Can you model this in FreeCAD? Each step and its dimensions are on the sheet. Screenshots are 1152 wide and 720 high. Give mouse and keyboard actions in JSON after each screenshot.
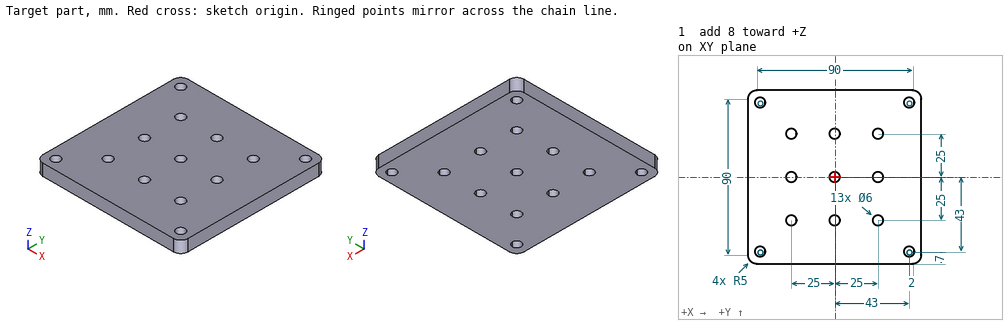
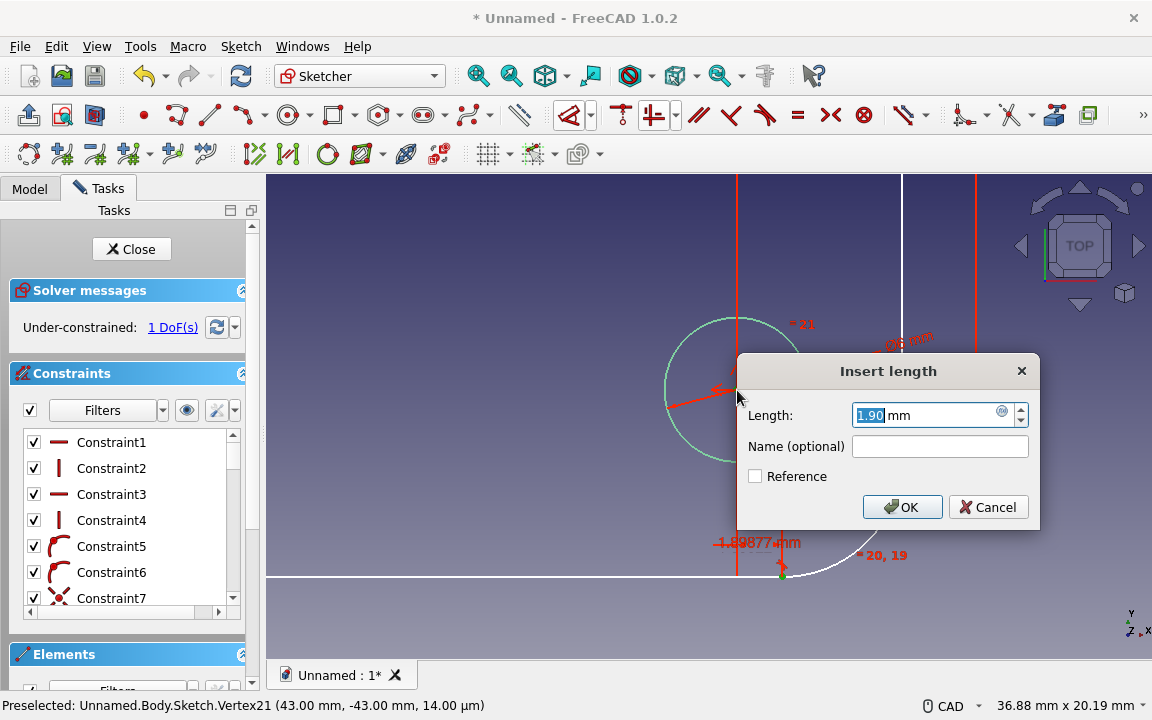
{"action": "type", "text": "2"}
{"action": "key", "text": "Return"}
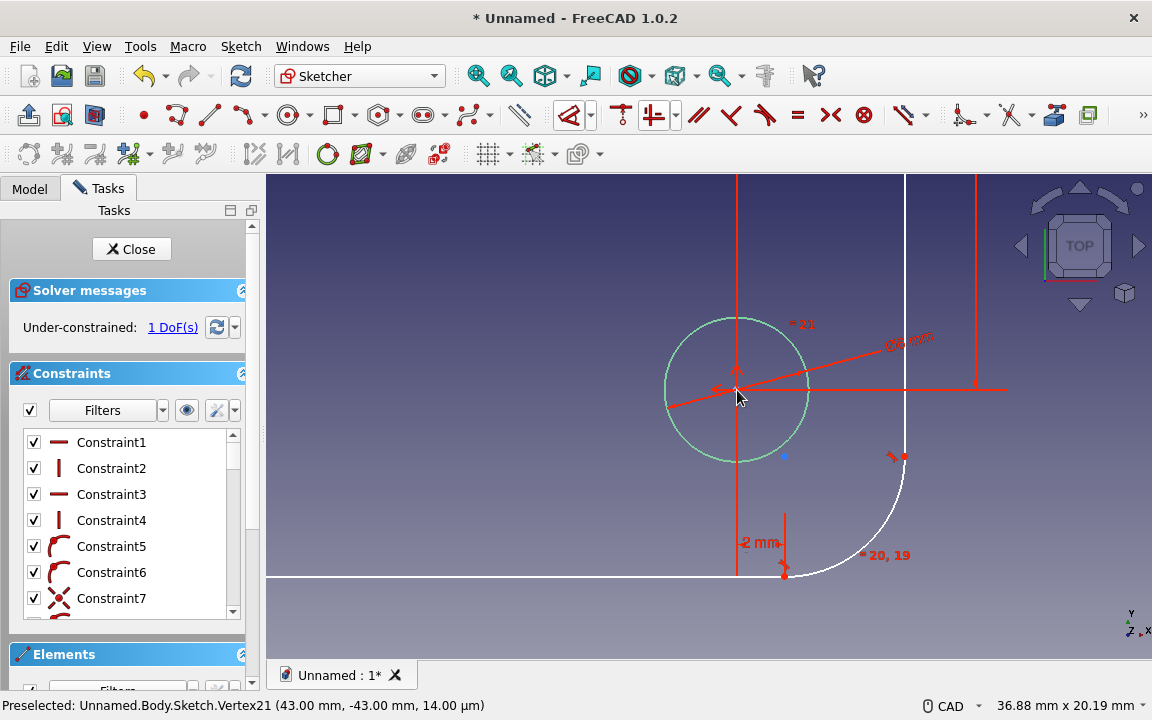
{"action": "scroll", "coordinate": [787, 582], "scroll_direction": "down", "scroll_amount": 10}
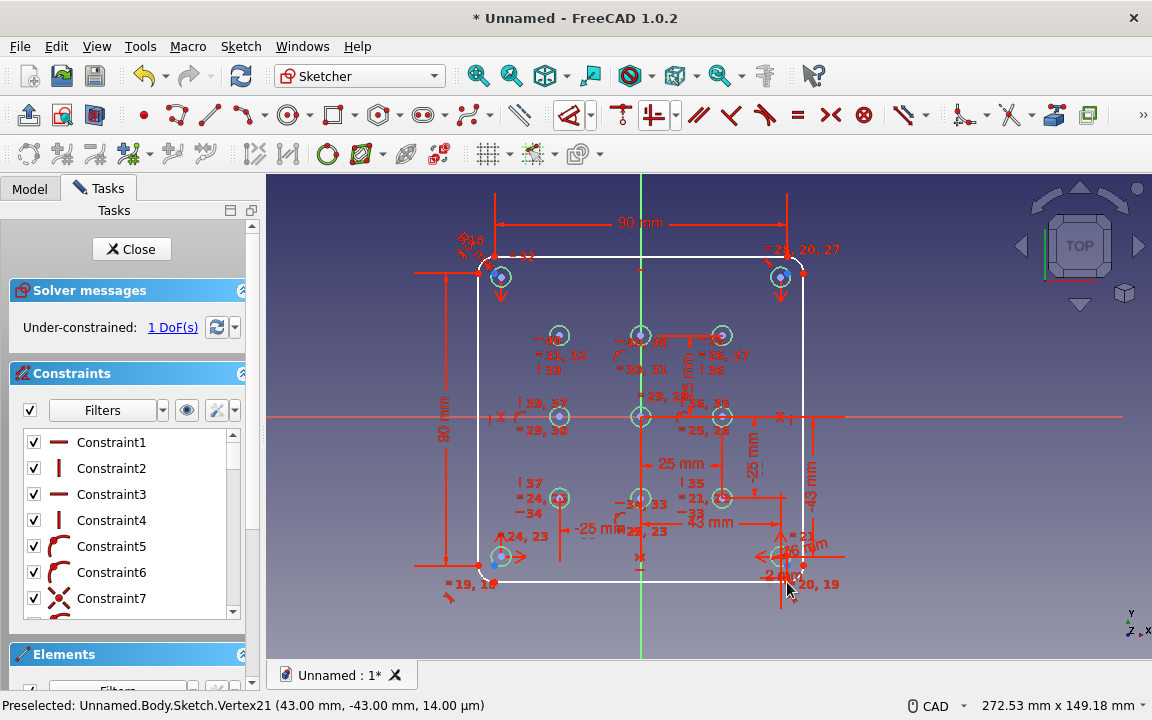
{"action": "scroll", "coordinate": [787, 582], "scroll_direction": "up", "scroll_amount": 3}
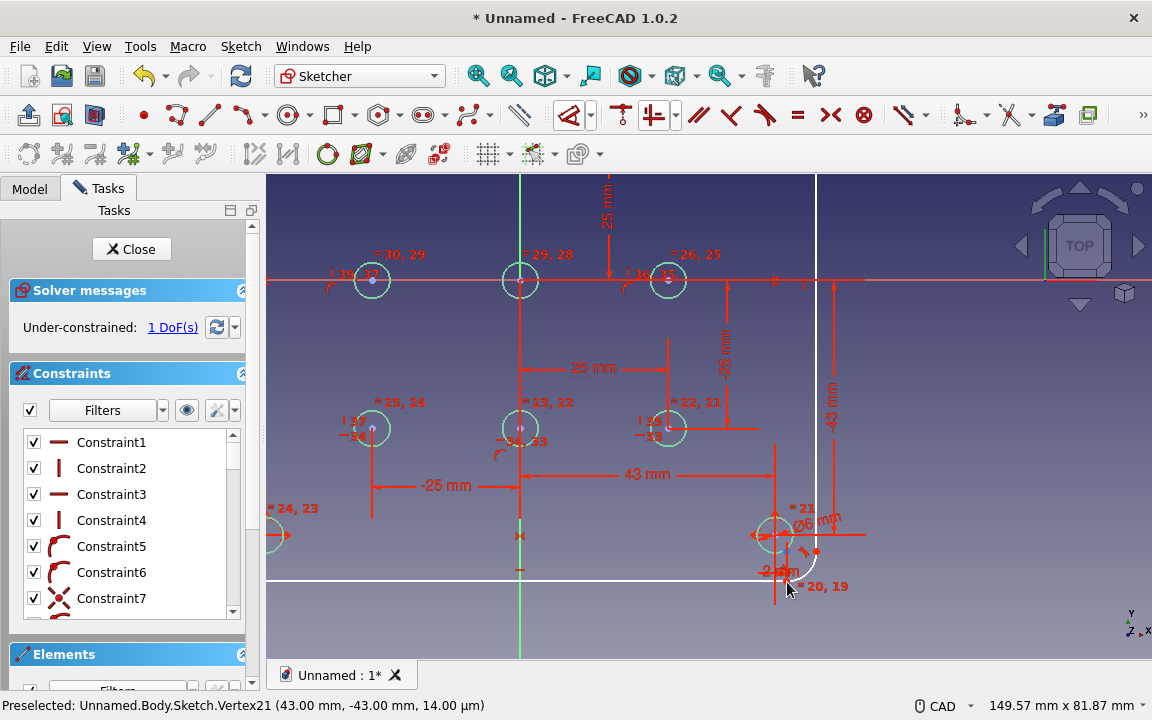
{"action": "left_click", "coordinate": [787, 581]}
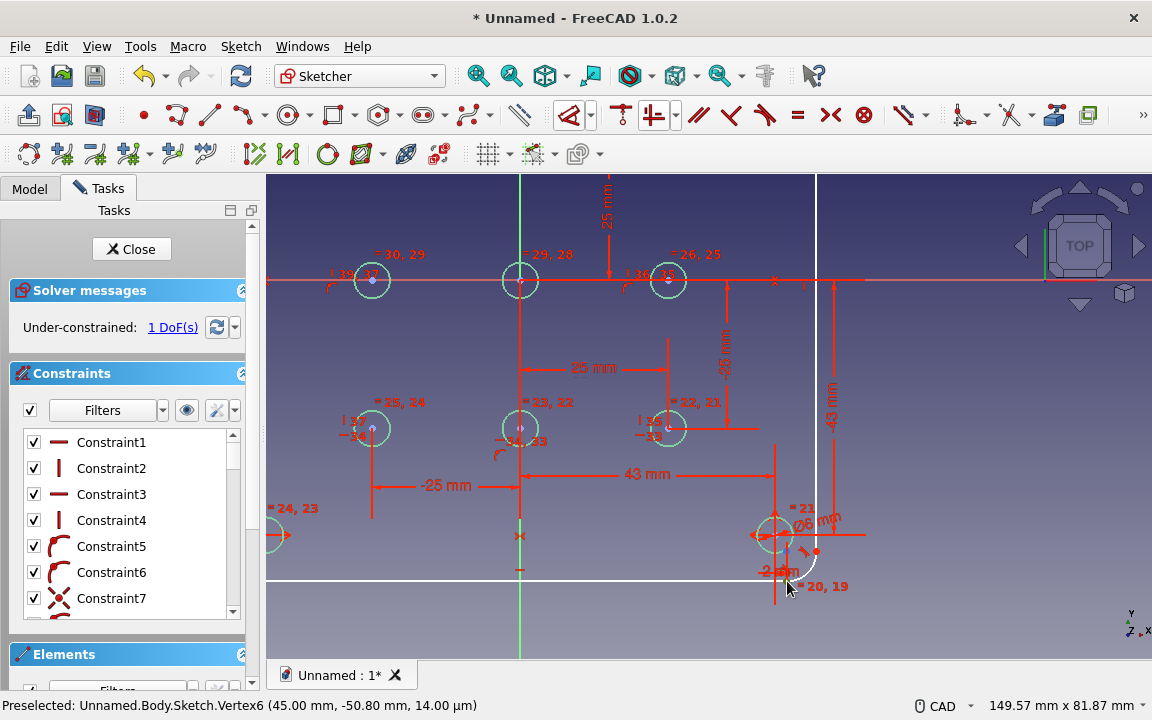
{"action": "left_click", "coordinate": [775, 535]}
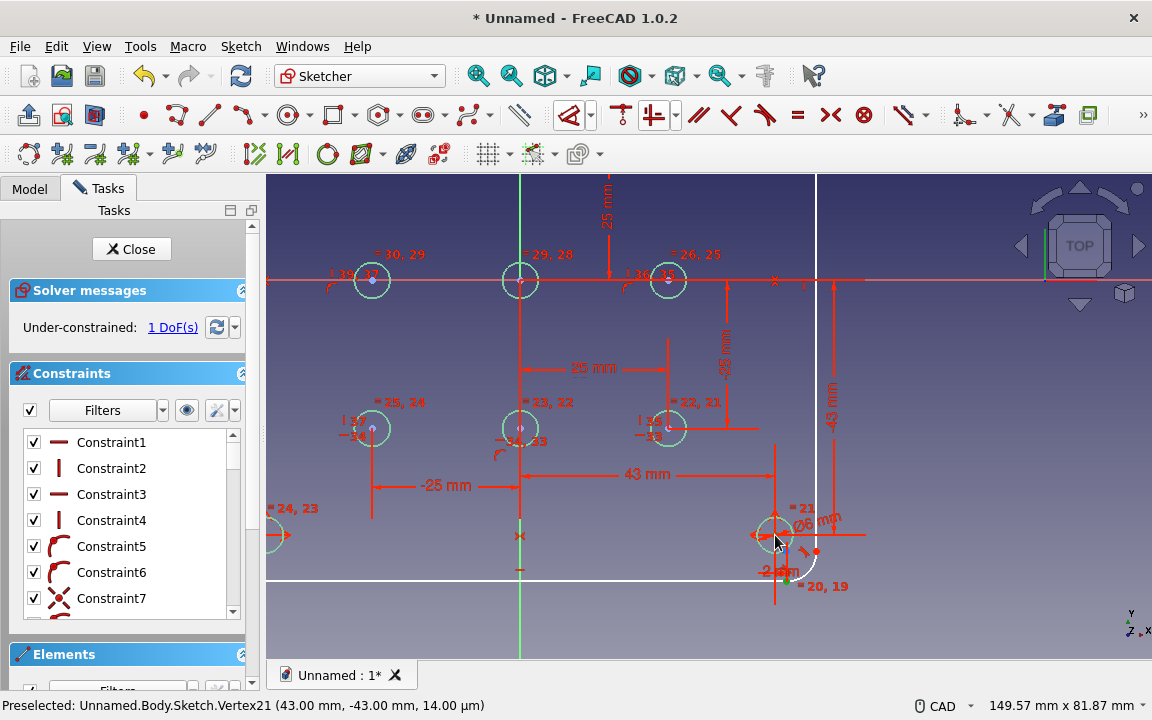
{"action": "left_click", "coordinate": [590, 116]}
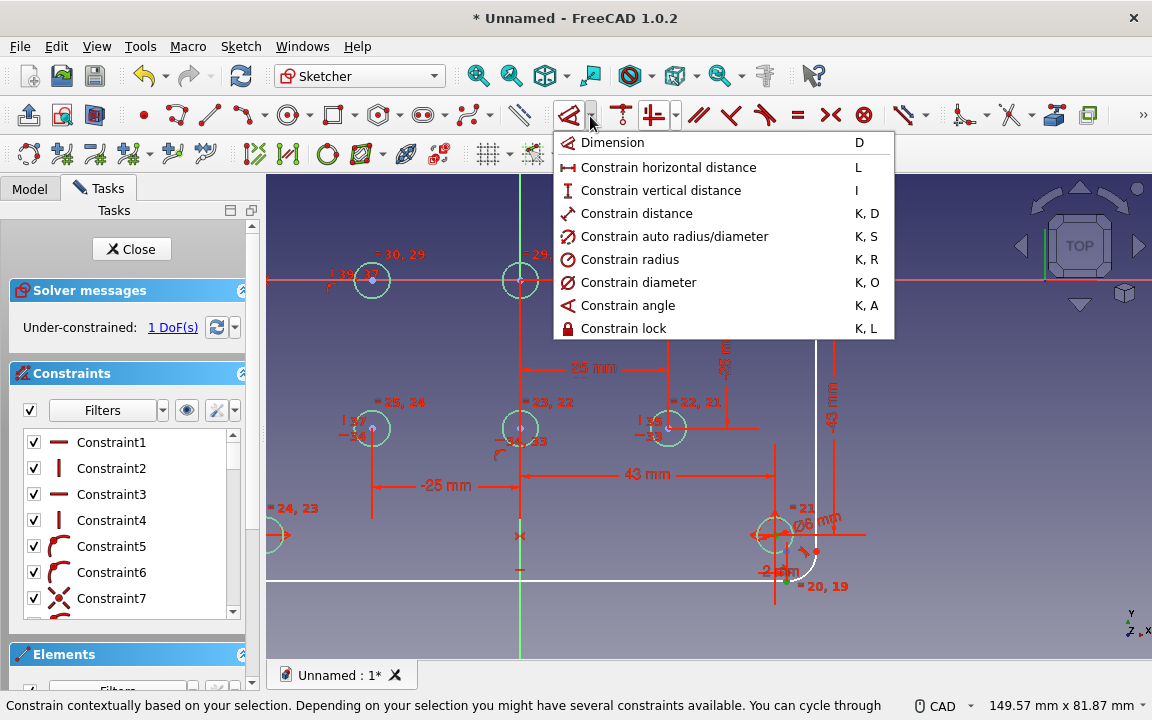
{"action": "left_click", "coordinate": [724, 190]}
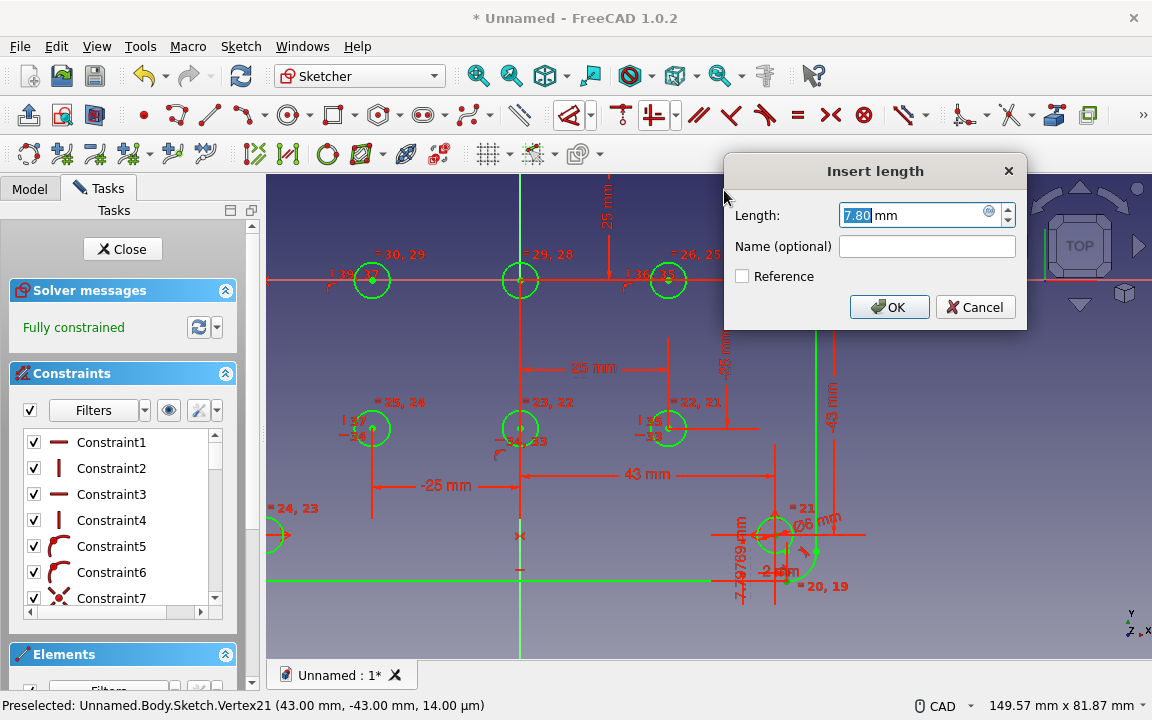
{"action": "type", "text": "7"}
{"action": "key", "text": "Return"}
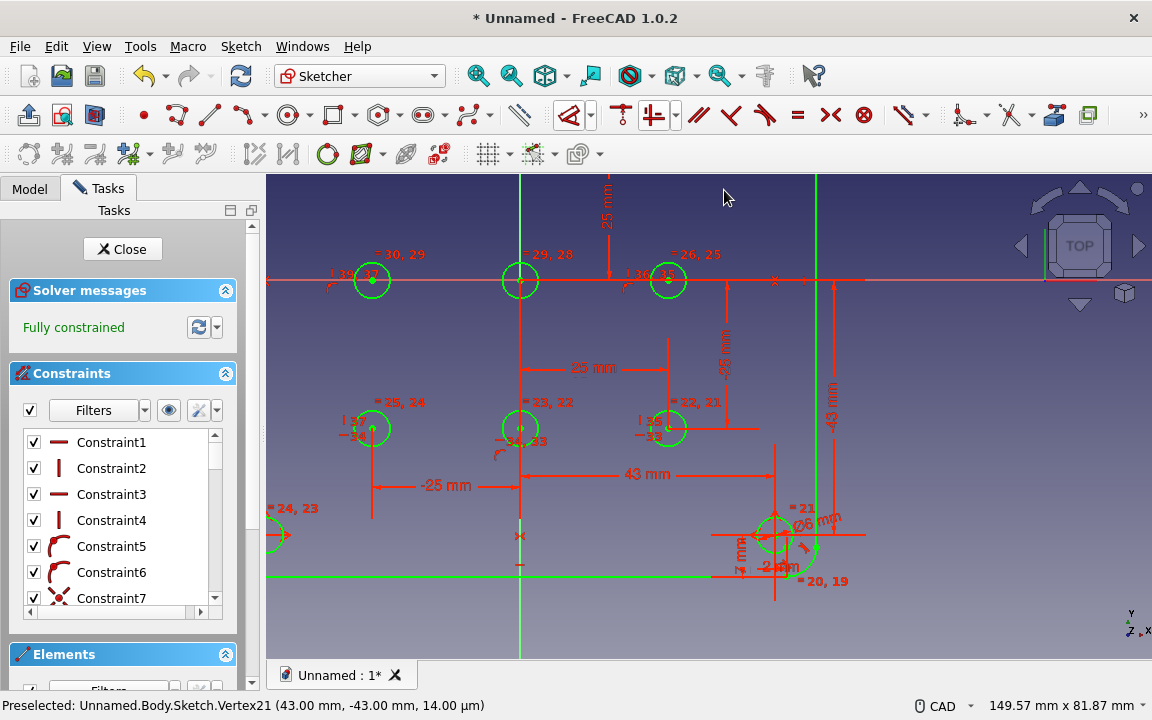
{"action": "left_click", "coordinate": [123, 249]}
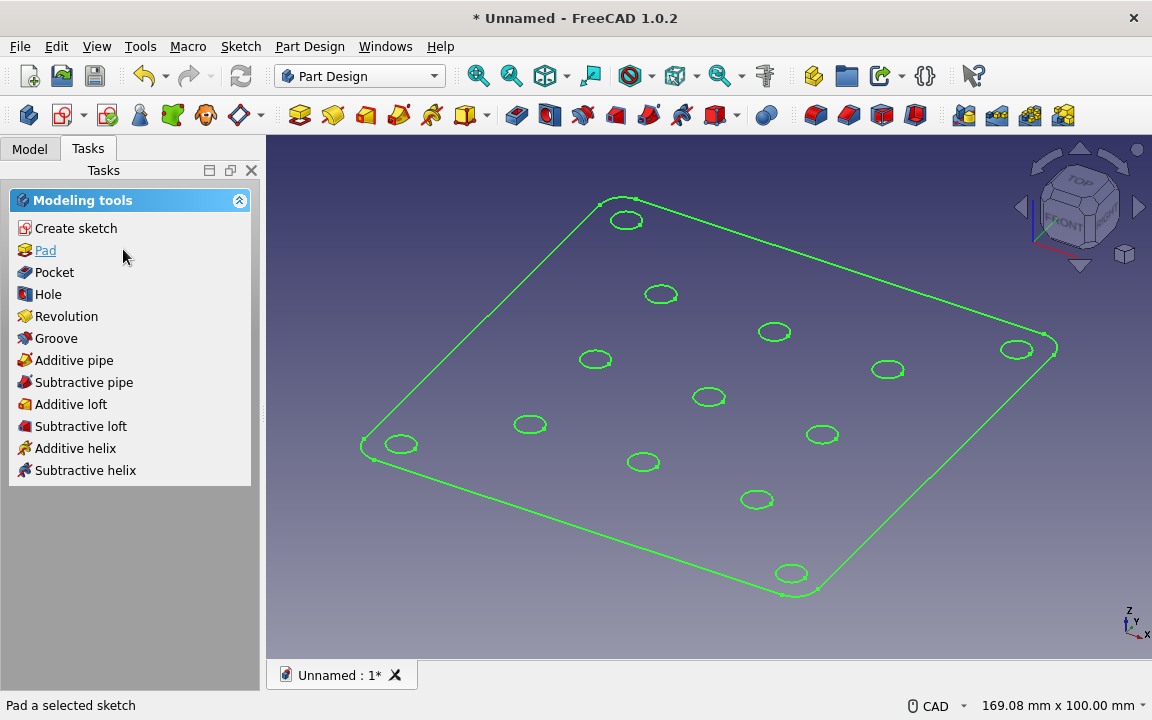
{"action": "left_click", "coordinate": [300, 116]}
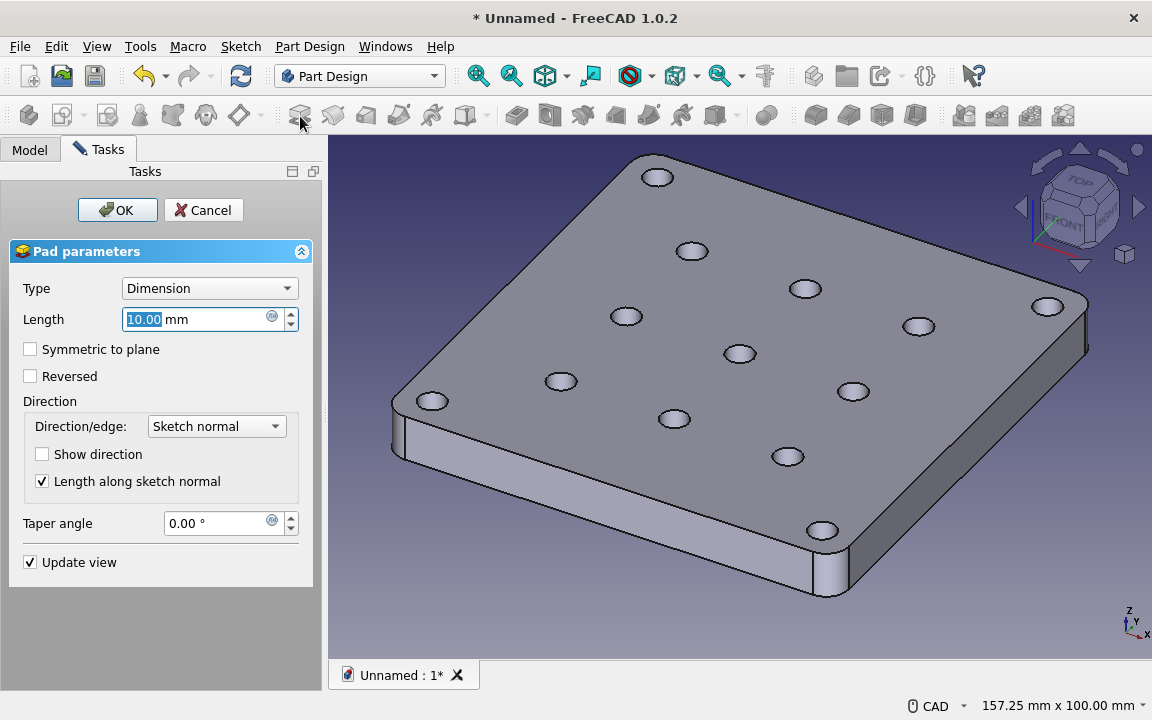
{"action": "type", "text": "8"}
{"action": "key", "text": "Tab"}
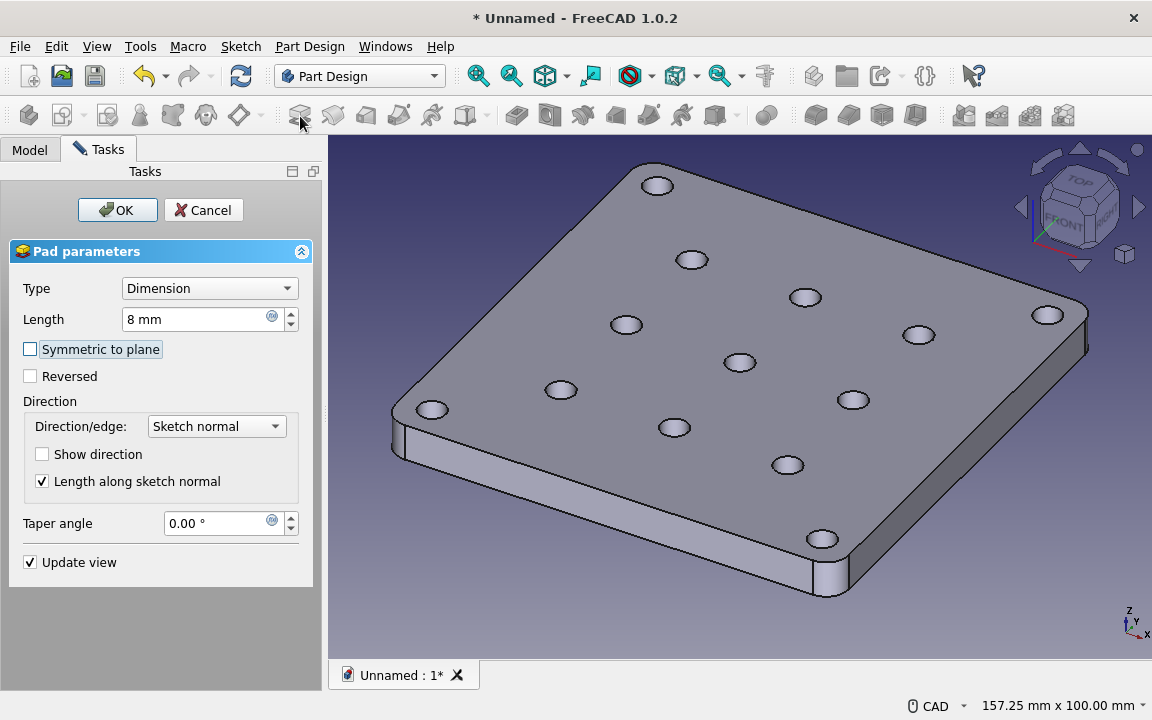
{"action": "left_click", "coordinate": [118, 210]}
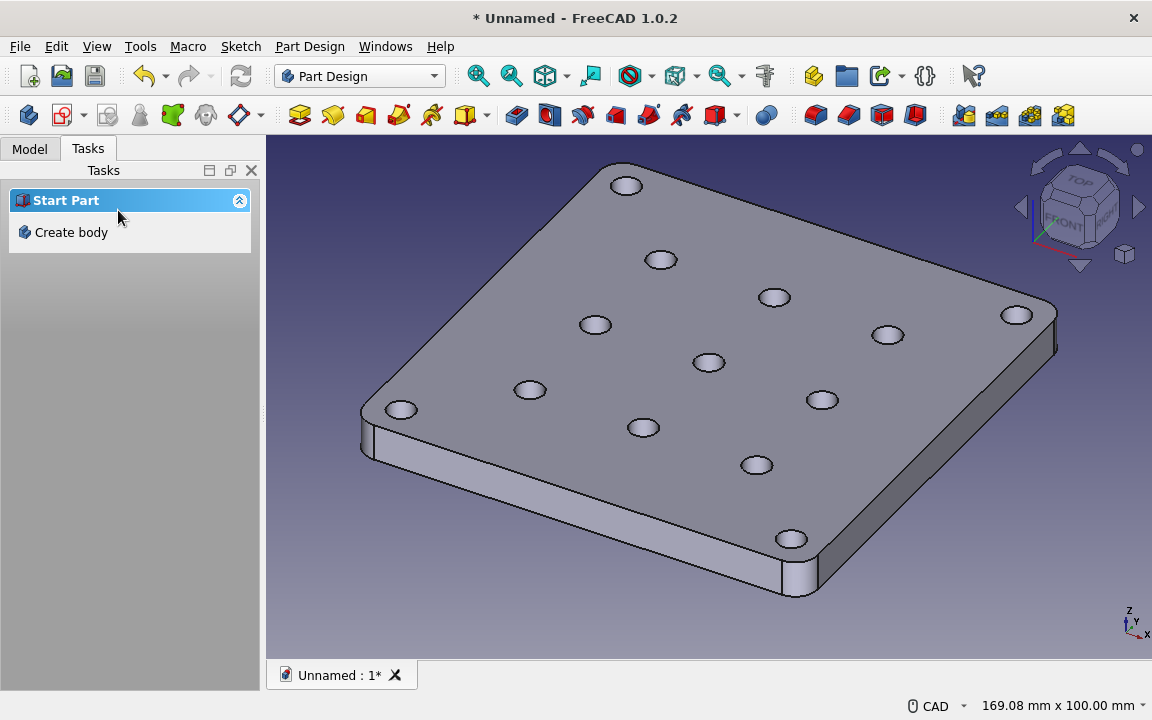
{"action": "key", "text": "0"}